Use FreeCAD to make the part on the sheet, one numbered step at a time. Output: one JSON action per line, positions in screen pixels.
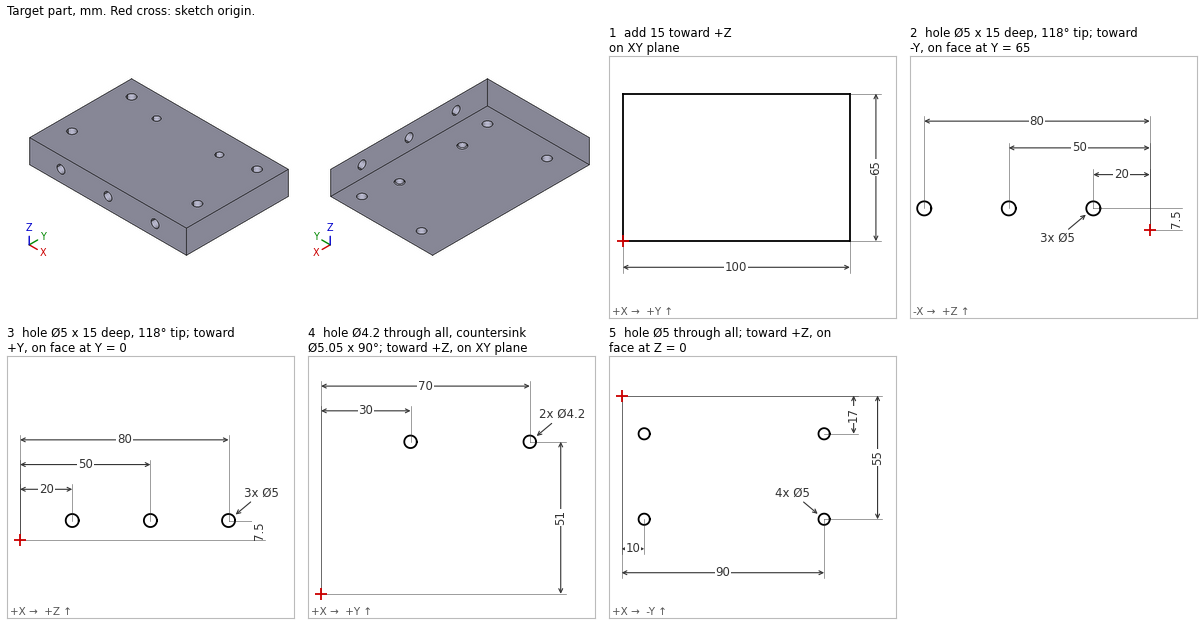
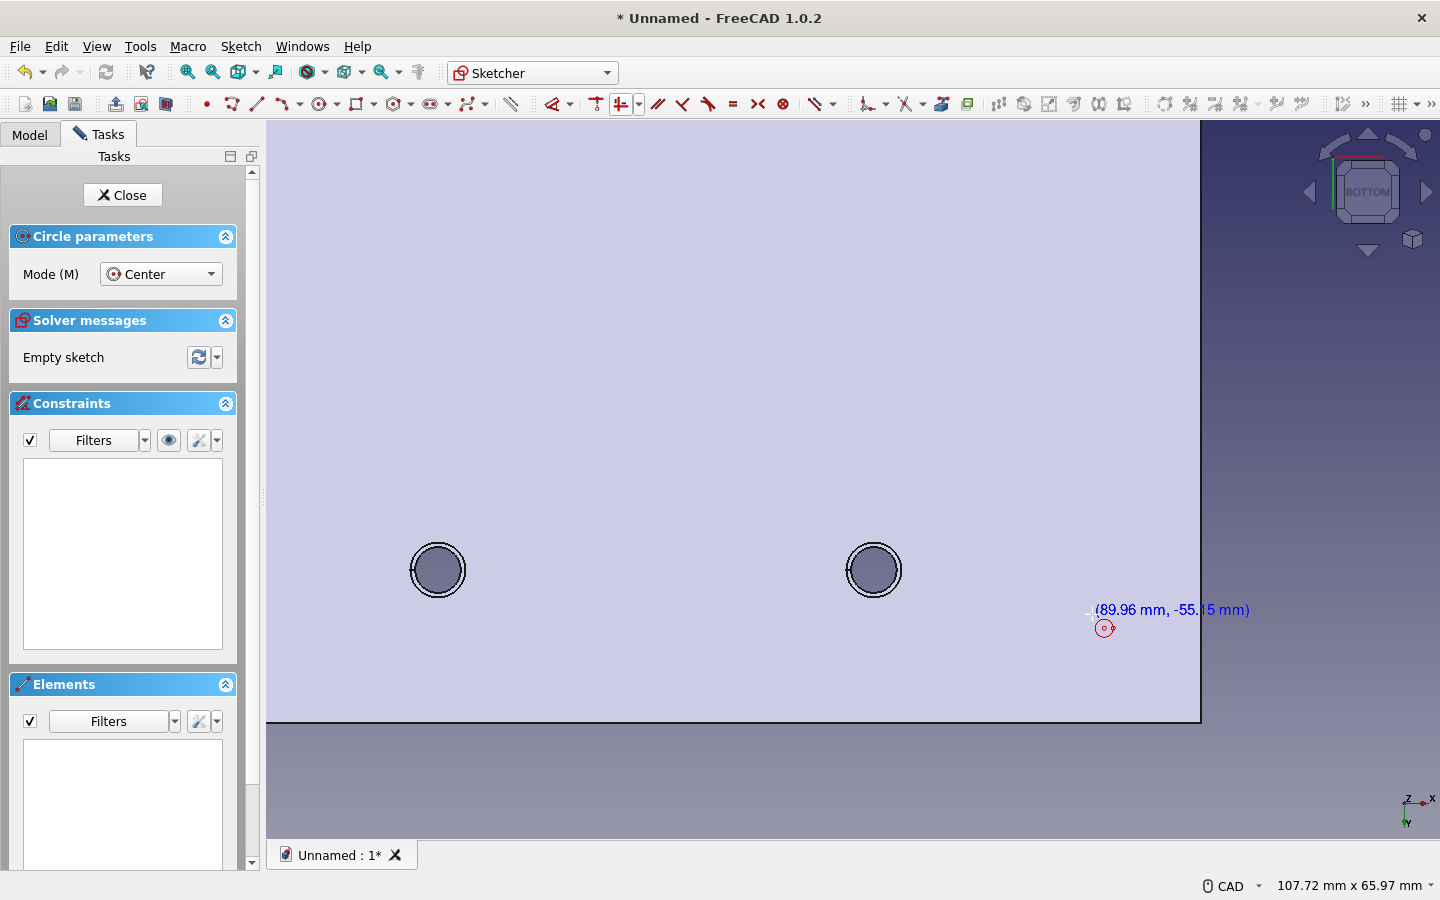
{"action": "left_click", "coordinate": [1092, 614]}
{"action": "mouse_move", "coordinate": [1111, 594]}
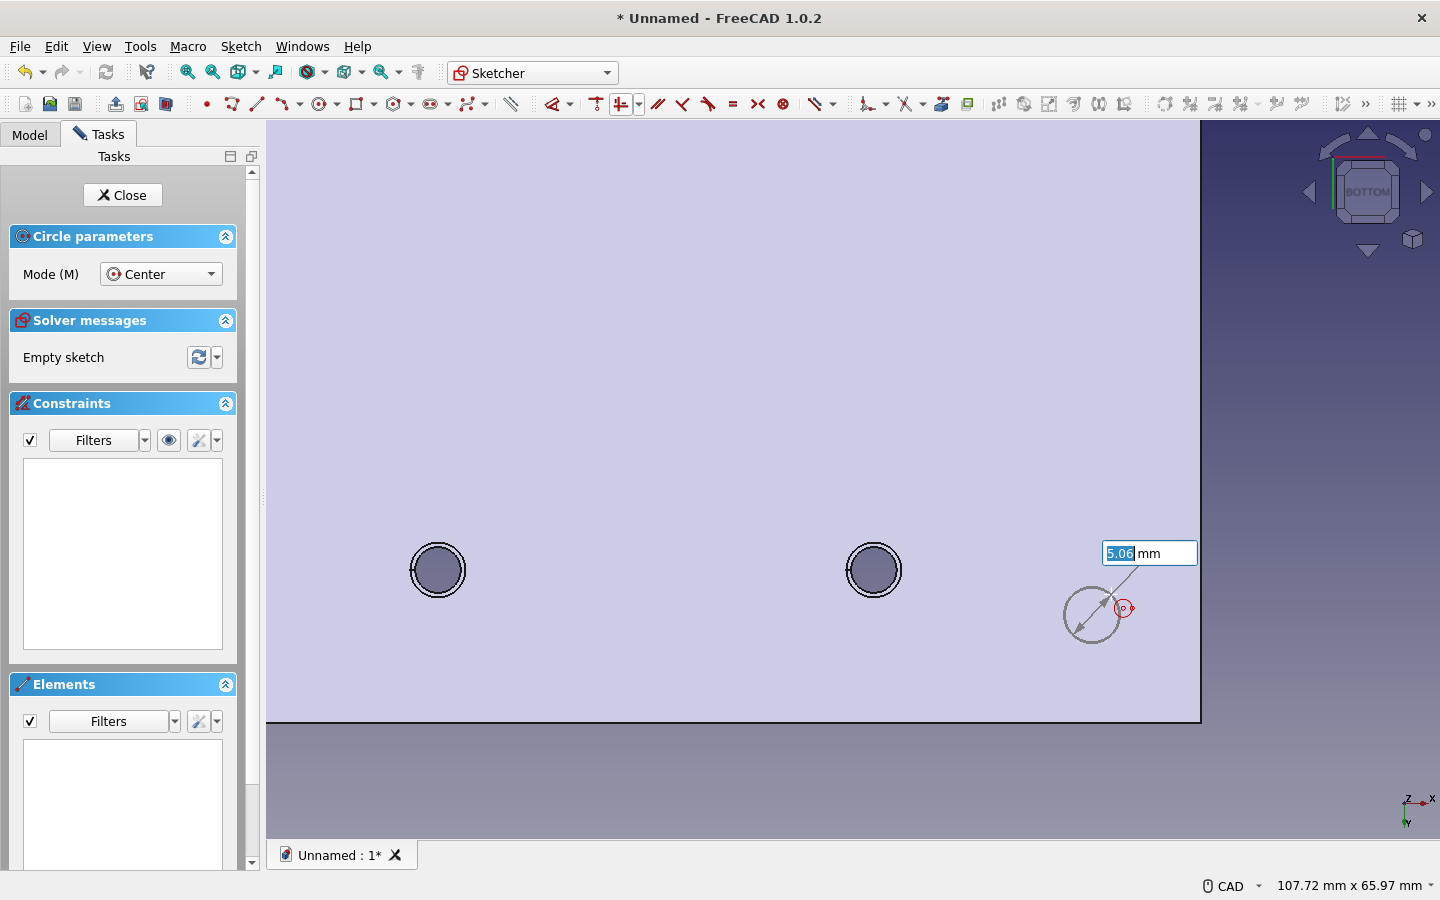
{"action": "type", "text": "5"}
{"action": "key", "text": "Return"}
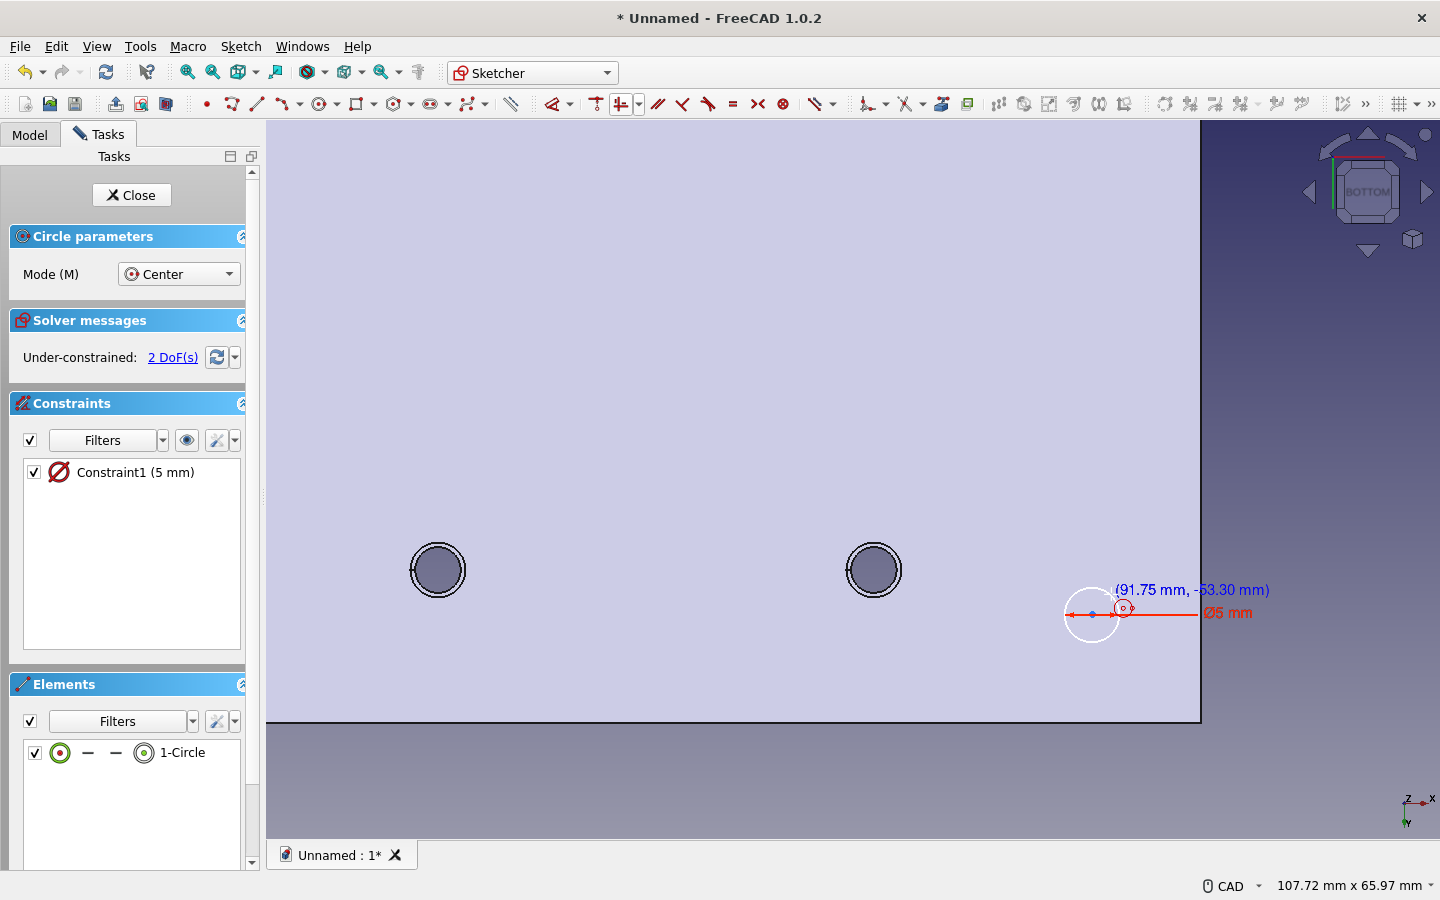
{"action": "scroll", "coordinate": [1129, 789], "scroll_direction": "down", "scroll_amount": 2}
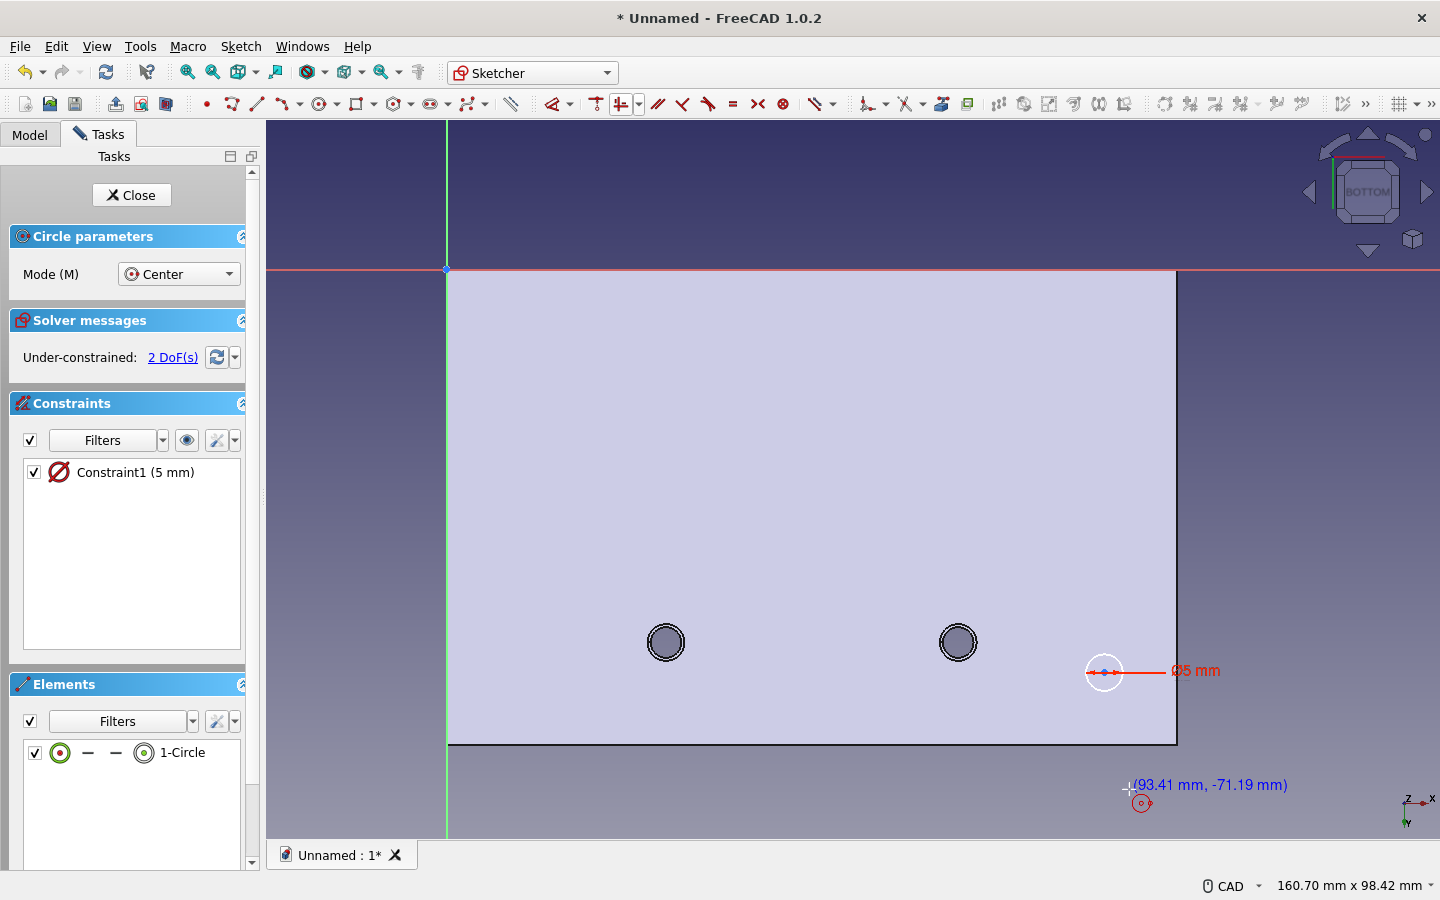
{"action": "scroll", "coordinate": [520, 672], "scroll_direction": "up", "scroll_amount": 2}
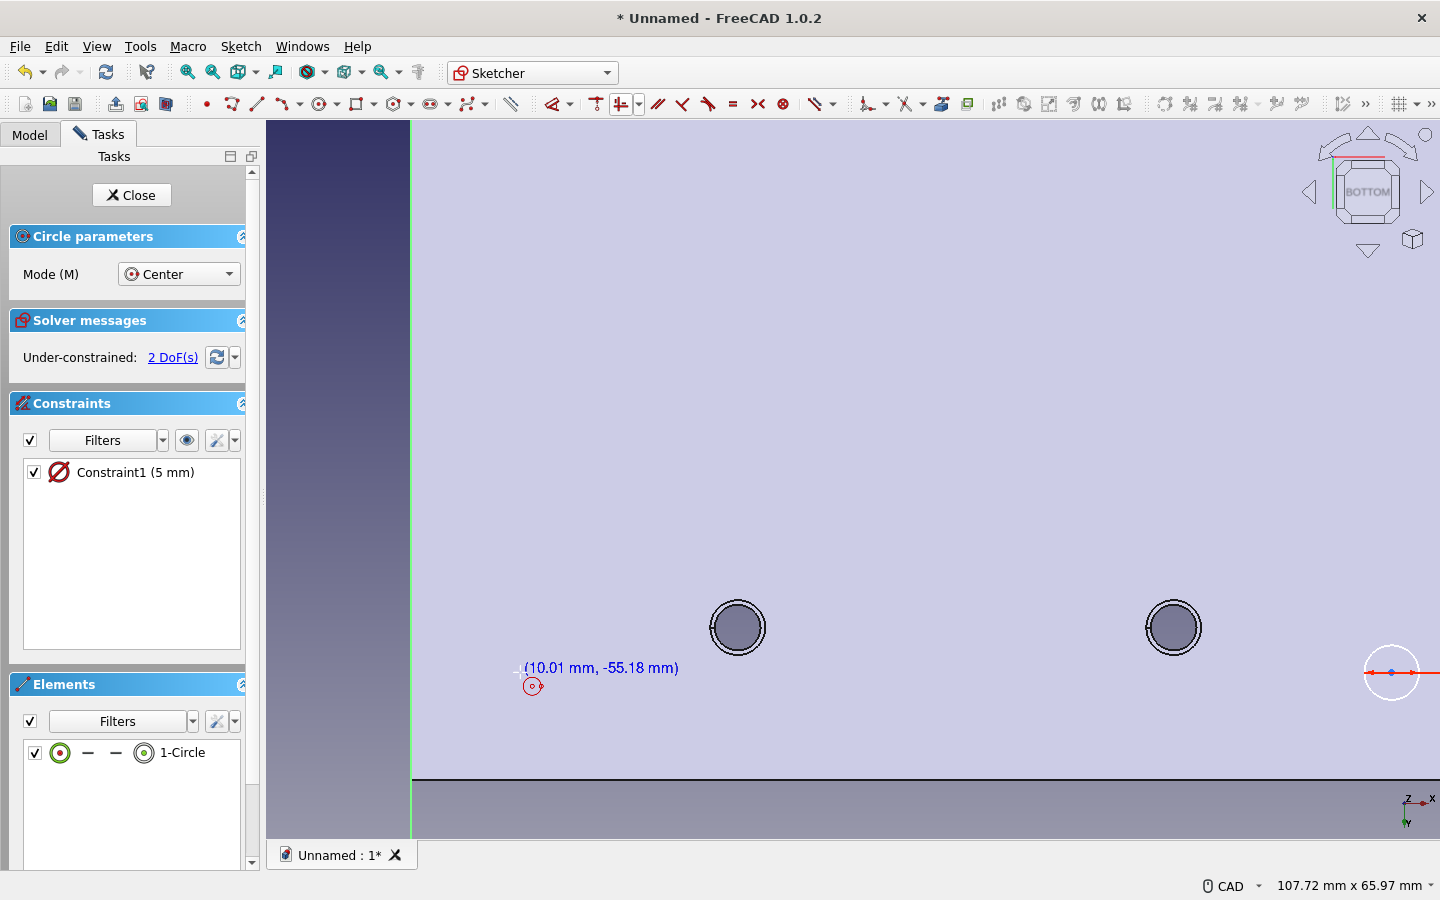
{"action": "left_click", "coordinate": [520, 671]}
{"action": "mouse_move", "coordinate": [539, 652]}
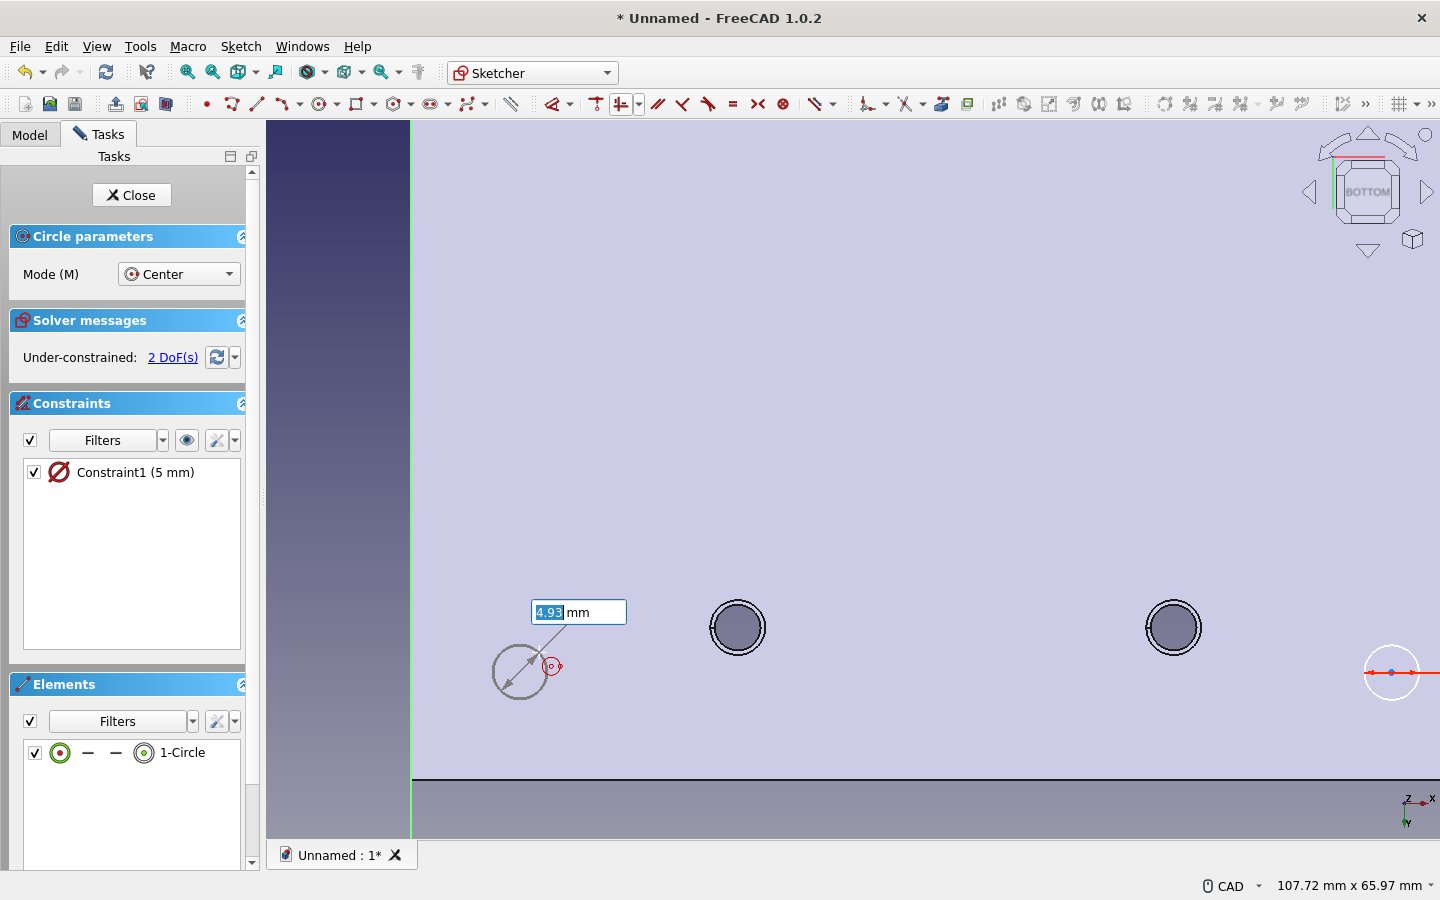
{"action": "type", "text": "5"}
{"action": "key", "text": "Return"}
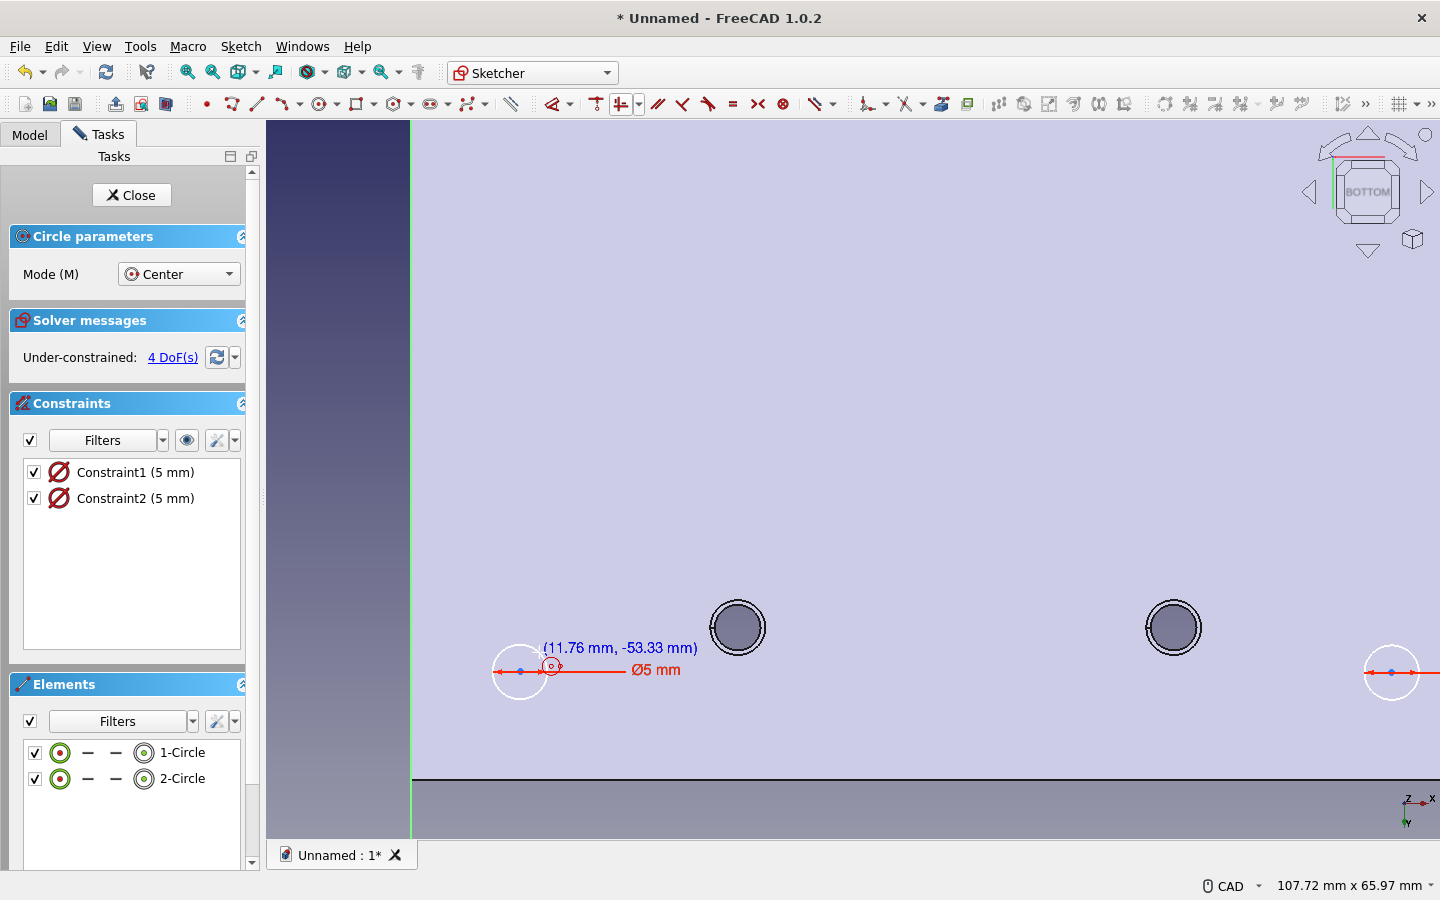
{"action": "scroll", "coordinate": [519, 671], "scroll_direction": "down", "scroll_amount": 2}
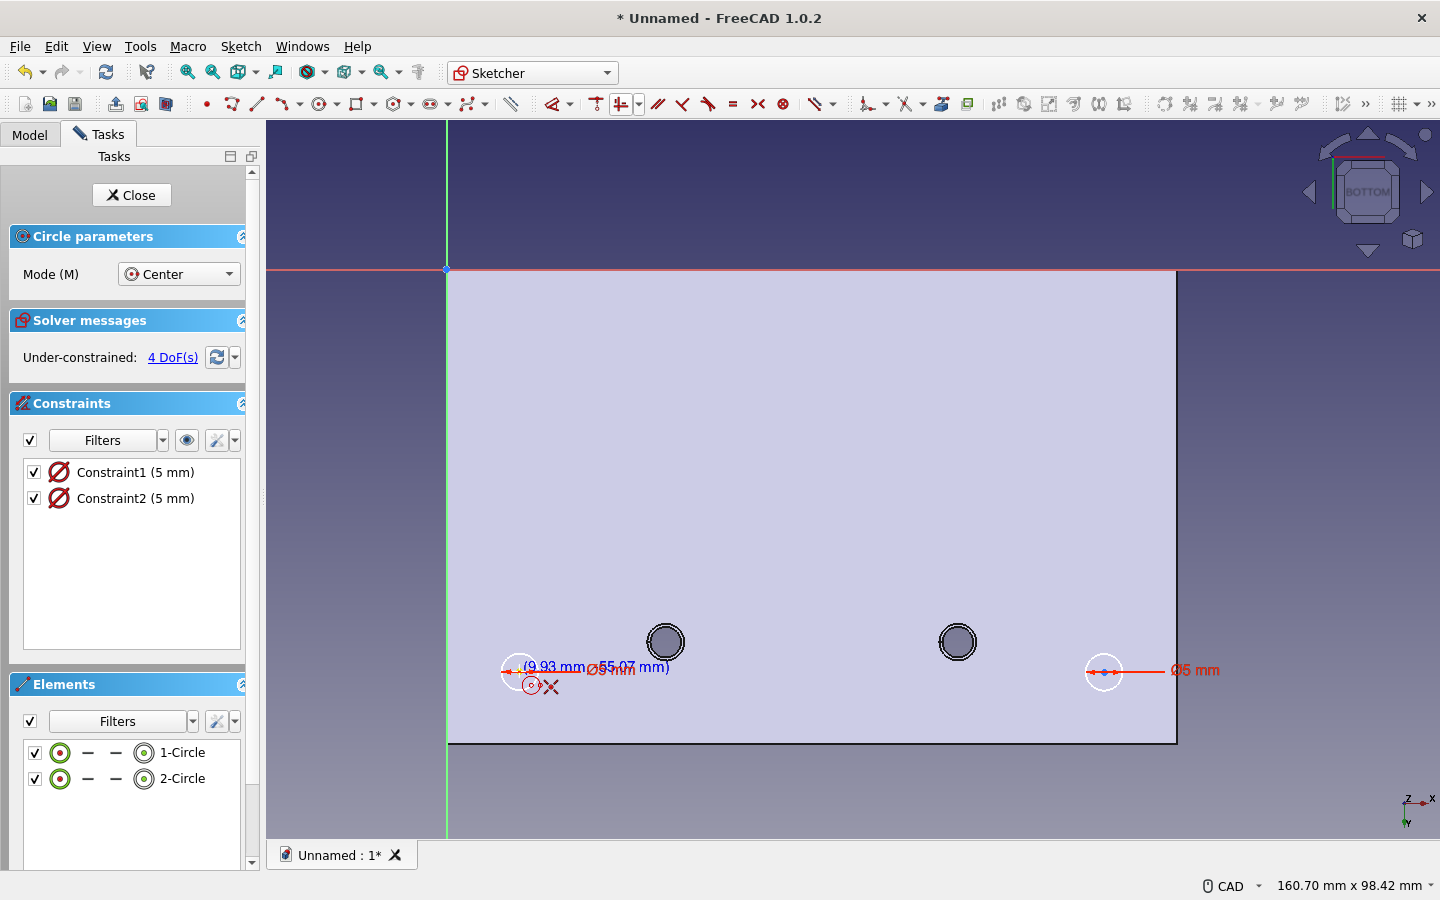
{"action": "scroll", "coordinate": [1104, 394], "scroll_direction": "up", "scroll_amount": 2}